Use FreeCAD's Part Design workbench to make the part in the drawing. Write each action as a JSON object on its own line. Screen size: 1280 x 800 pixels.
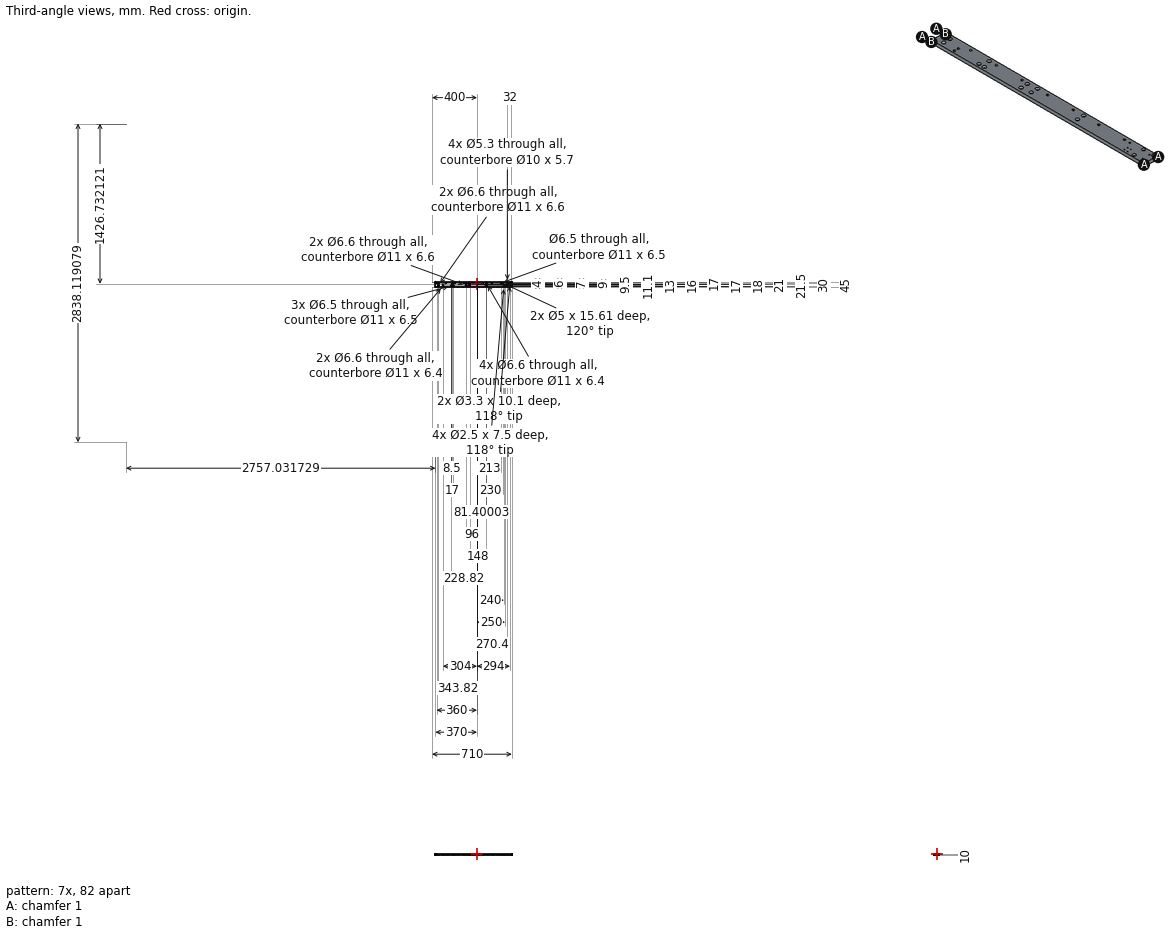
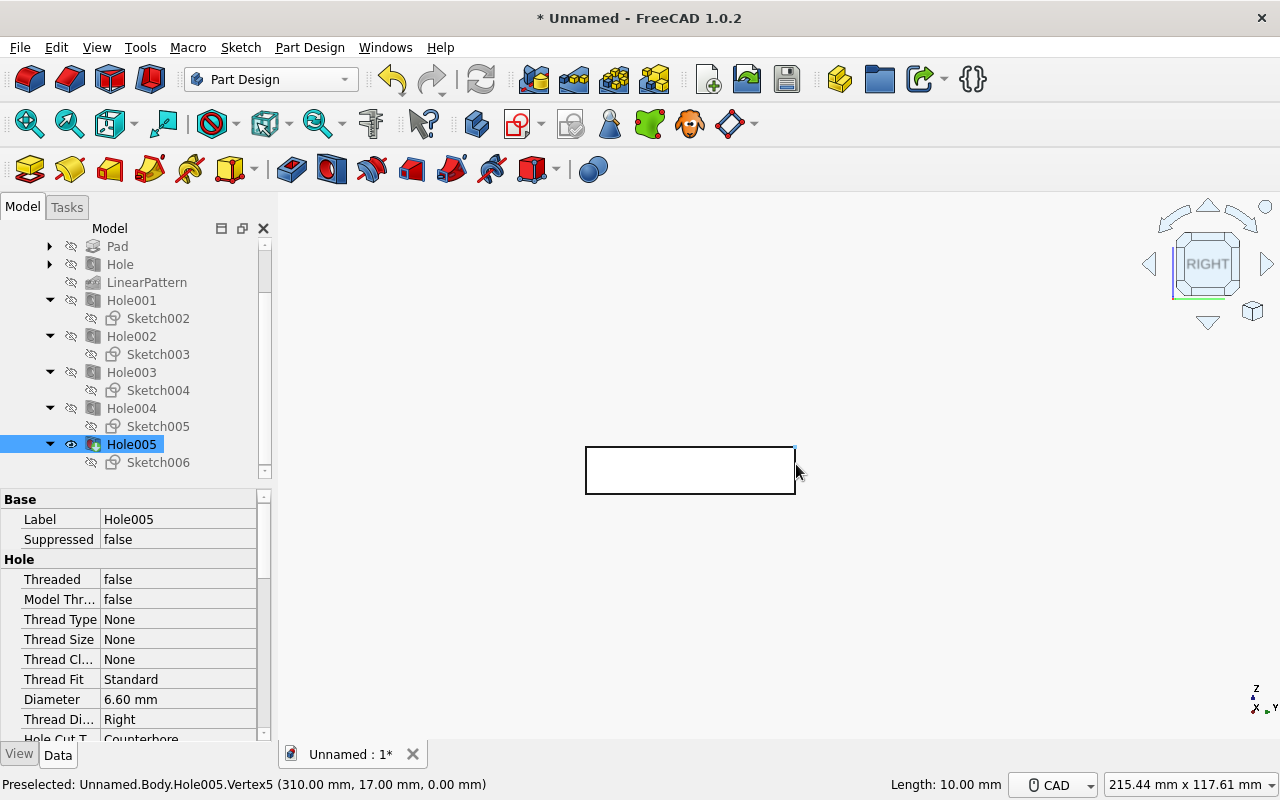
{"action": "left_click", "coordinate": [795, 470], "text": "ctrl"}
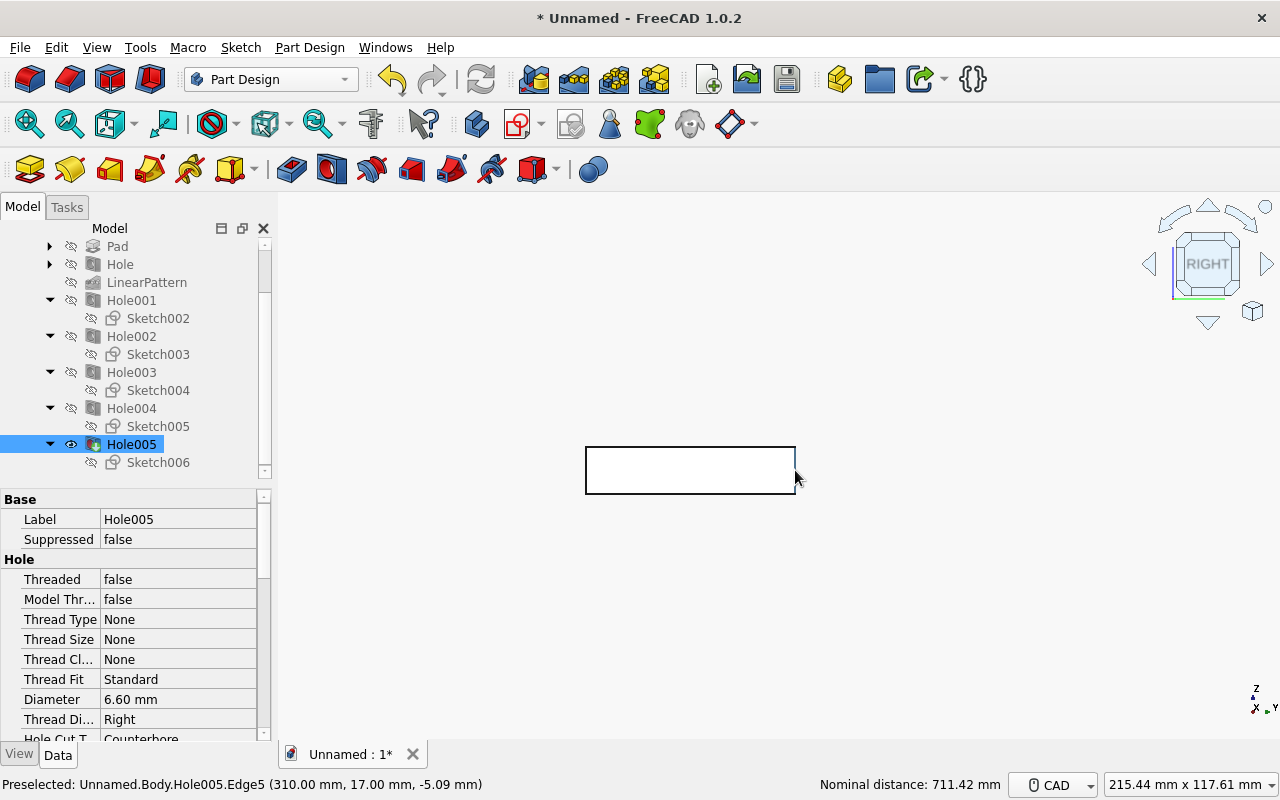
{"action": "left_click", "coordinate": [586, 470], "text": "ctrl"}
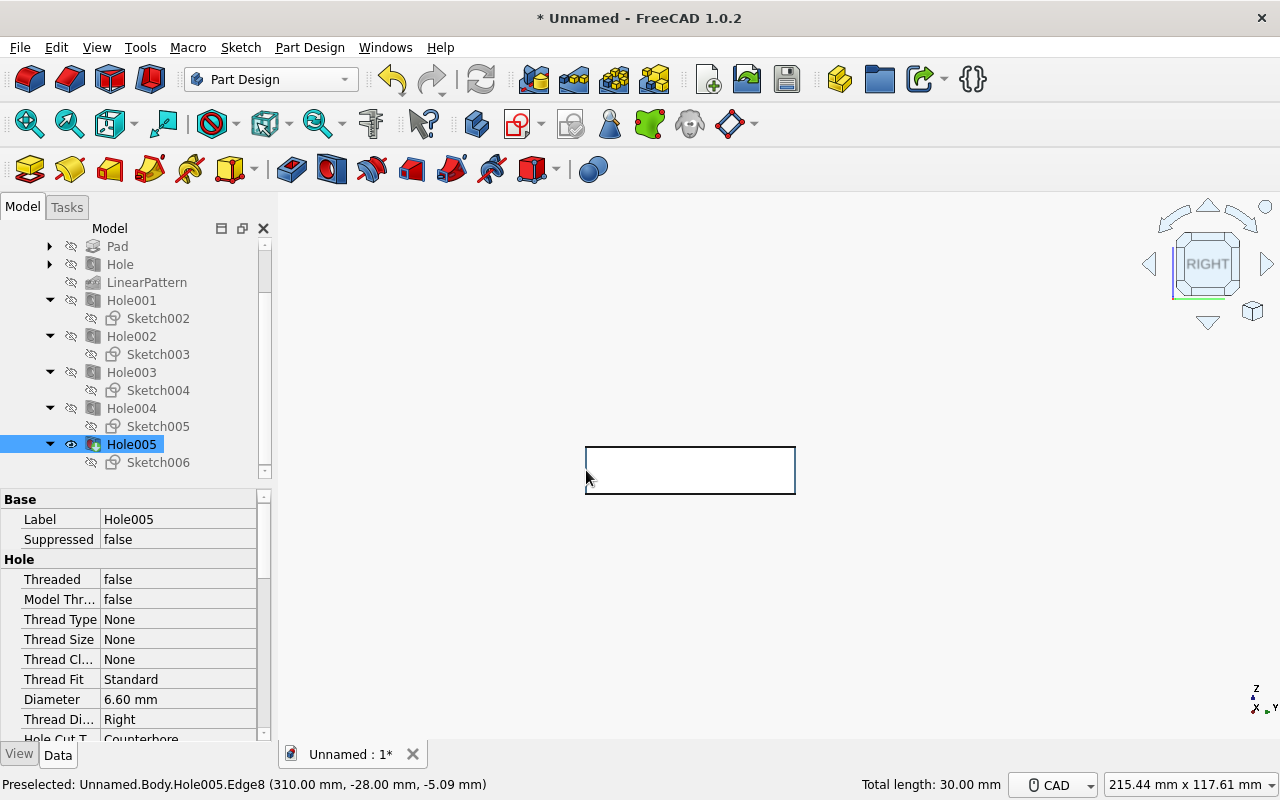
{"action": "left_click", "coordinate": [30, 124]}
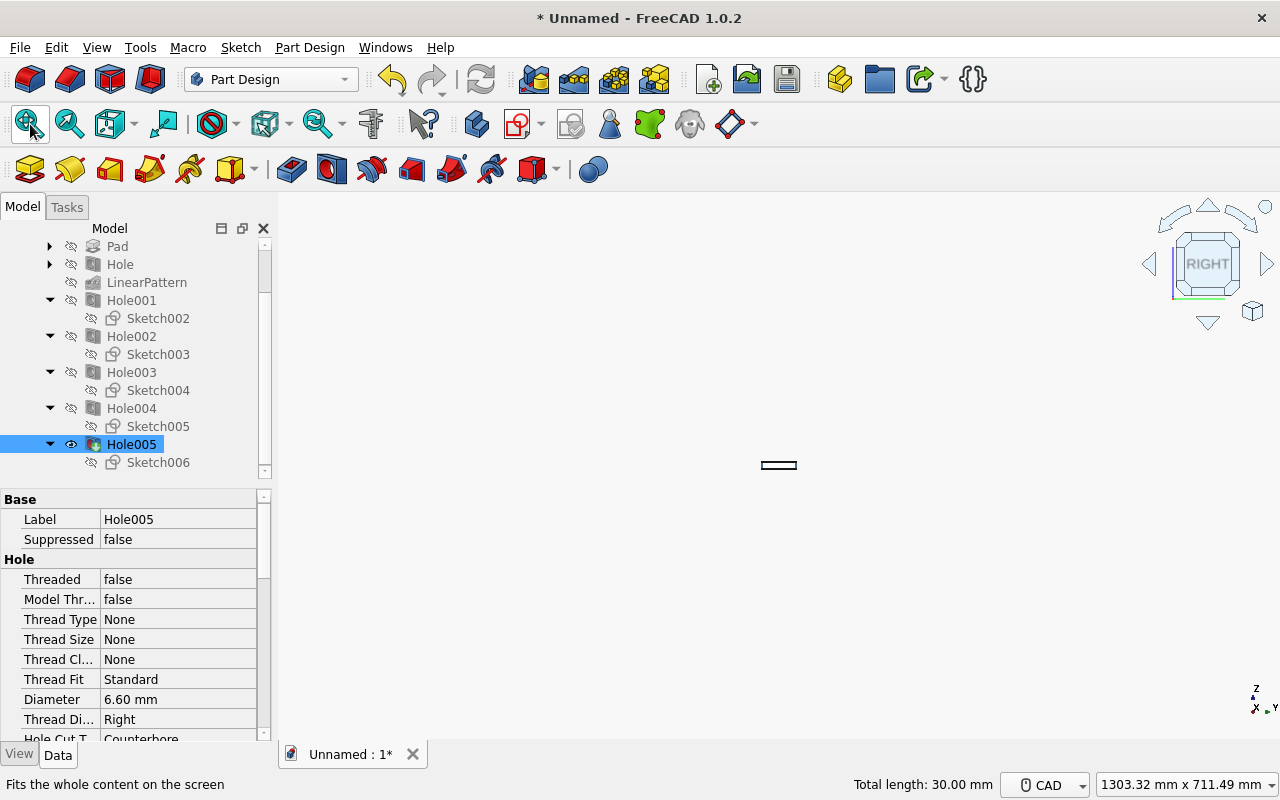
{"action": "key", "text": "5"}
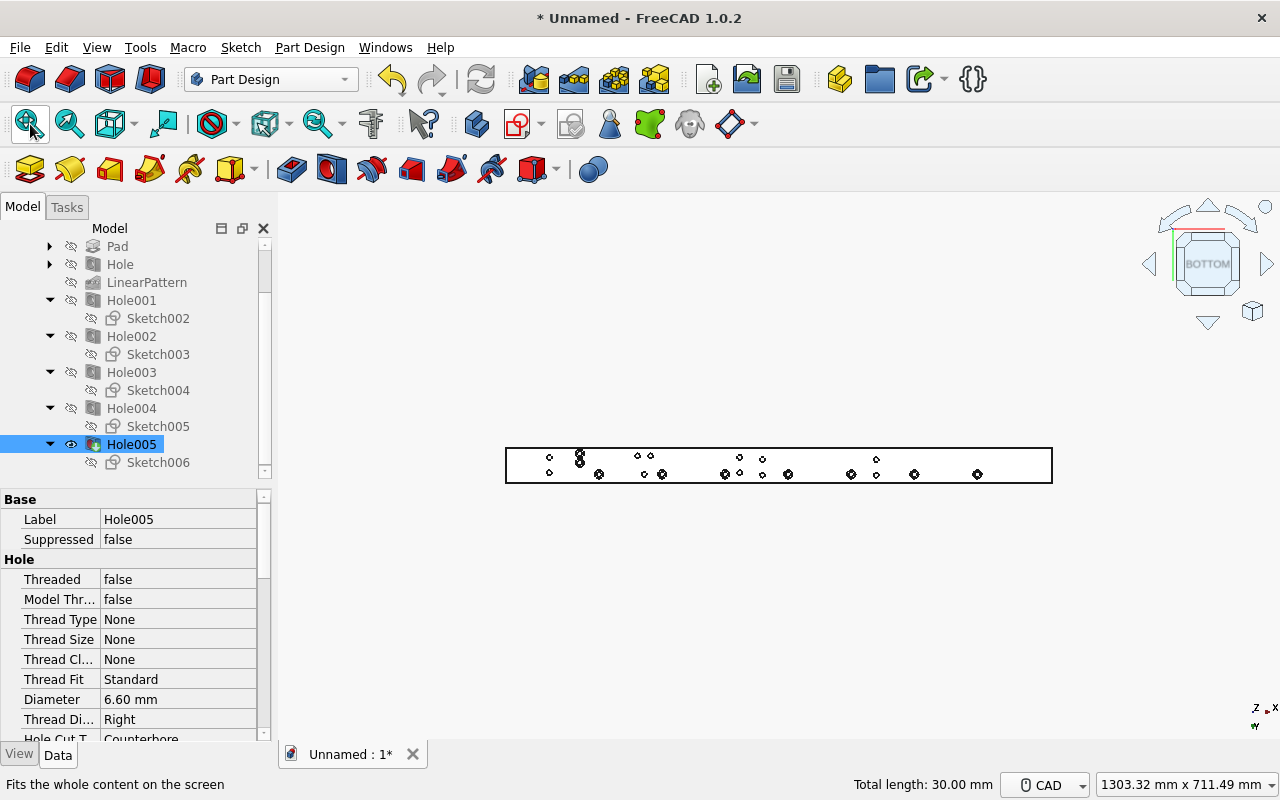
{"action": "scroll", "coordinate": [506, 482], "scroll_direction": "up", "scroll_amount": 9}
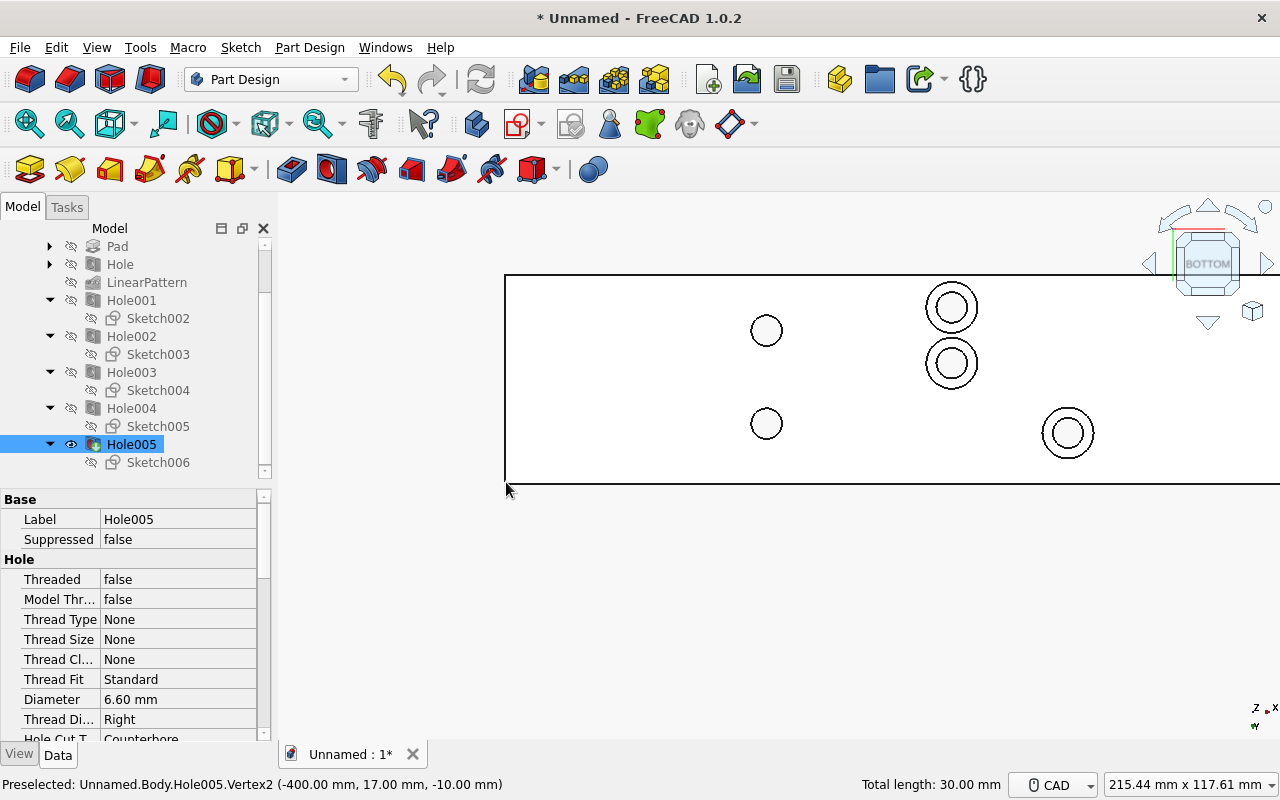
{"action": "left_click", "coordinate": [30, 124]}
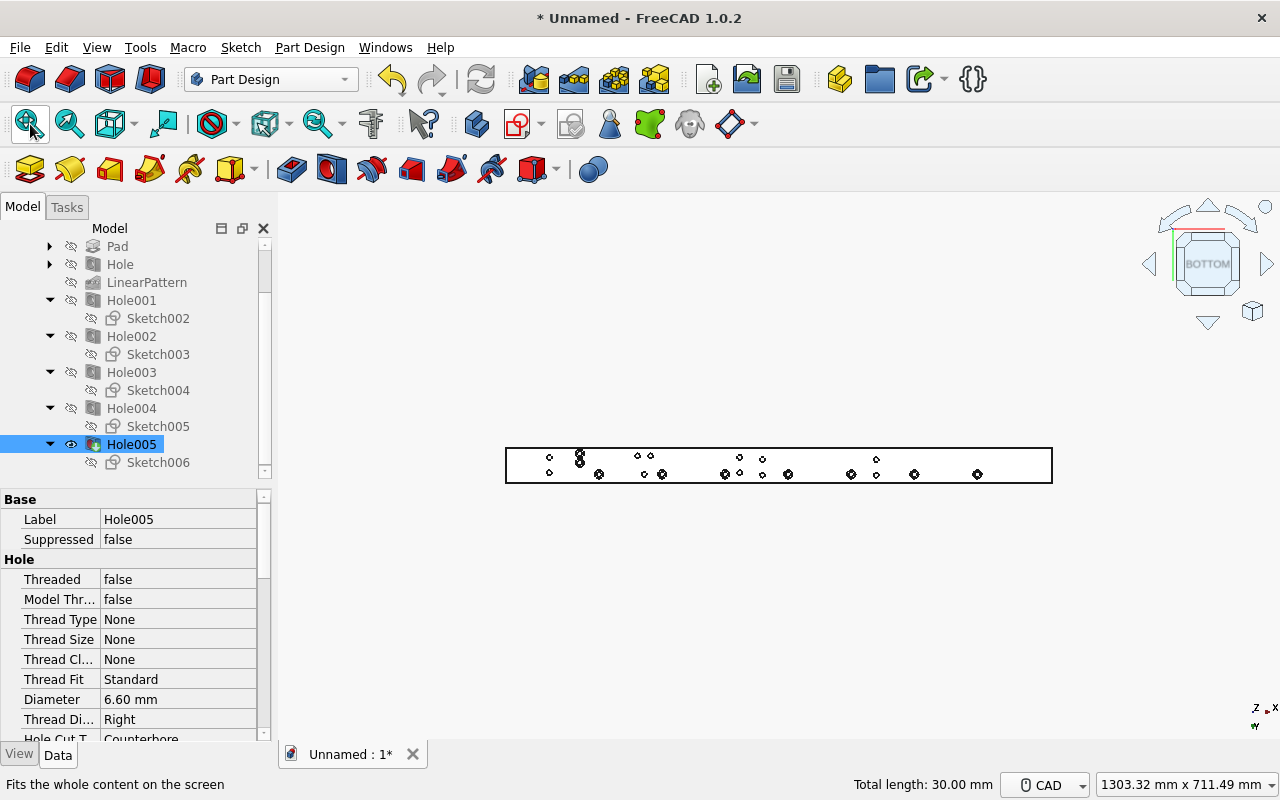
{"action": "key", "text": "4"}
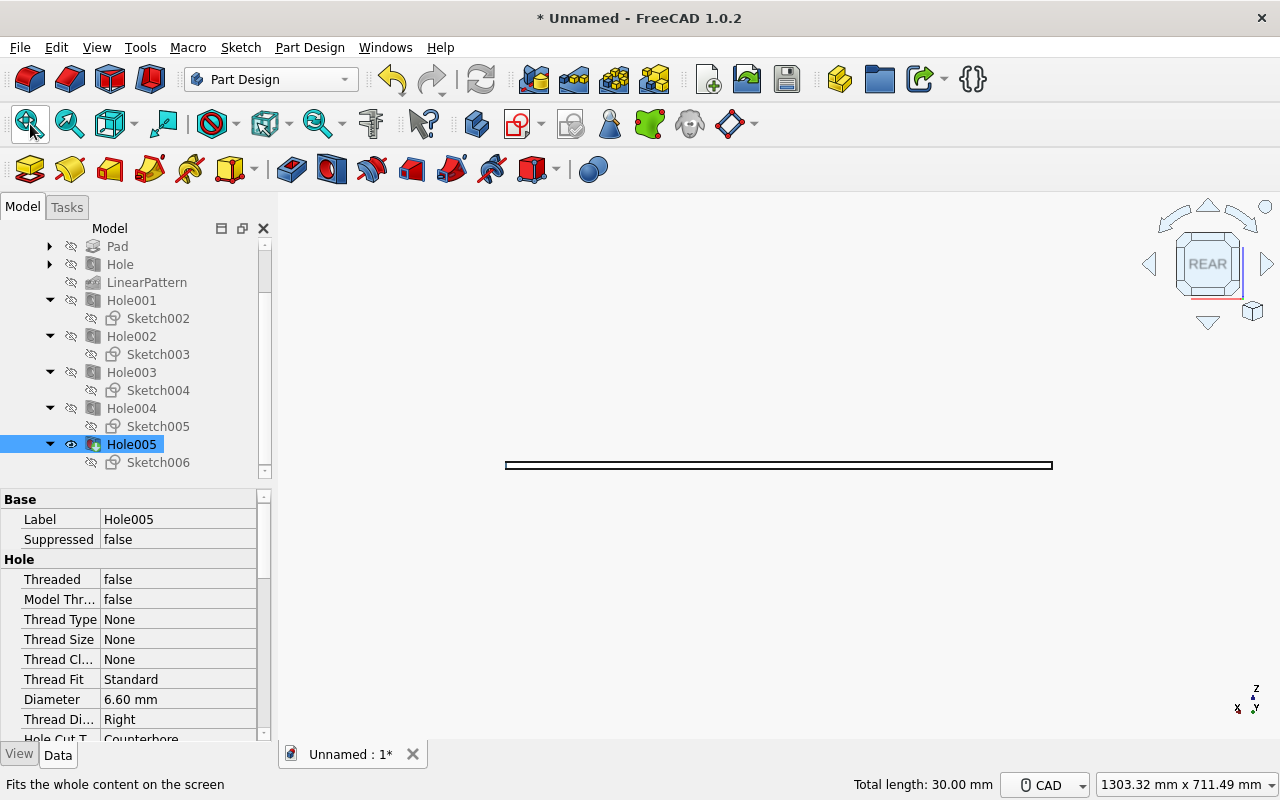
{"action": "scroll", "coordinate": [1052, 465], "scroll_direction": "up", "scroll_amount": 9}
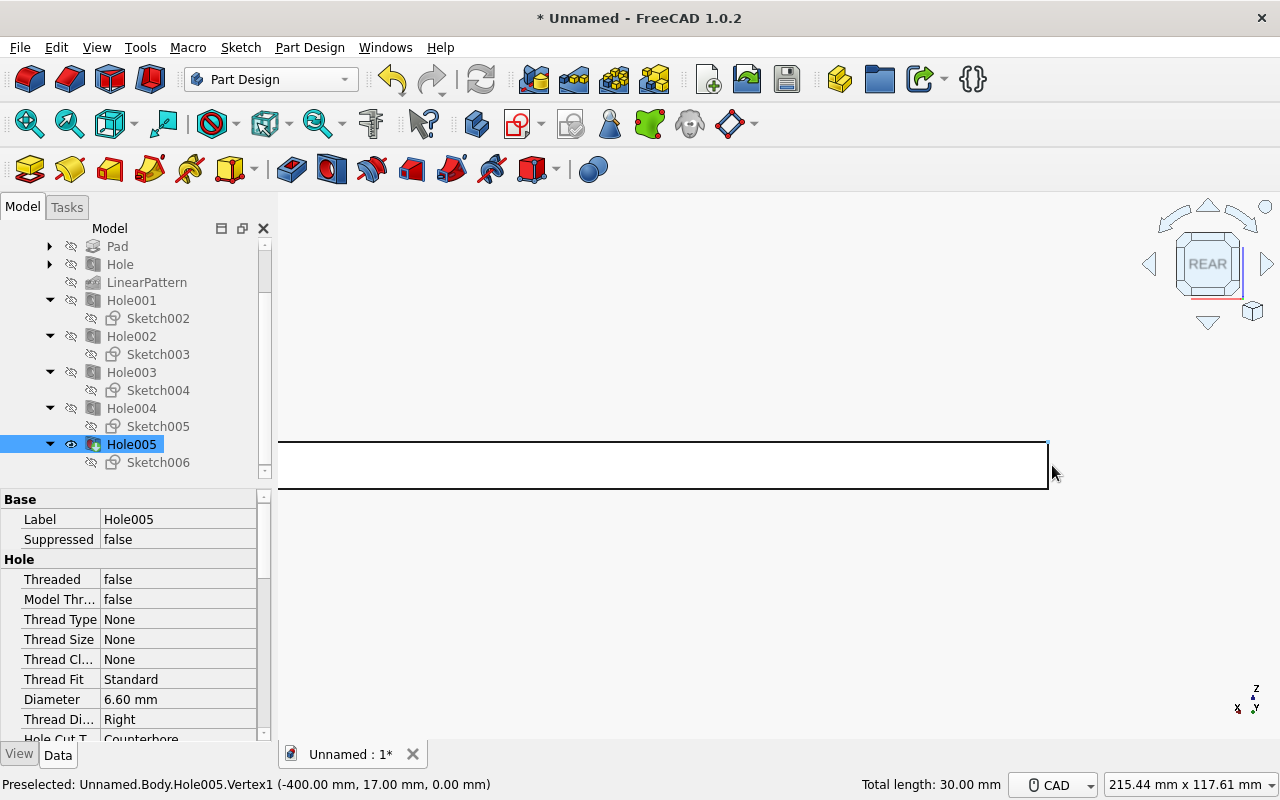
{"action": "left_click", "coordinate": [1048, 465], "text": "ctrl"}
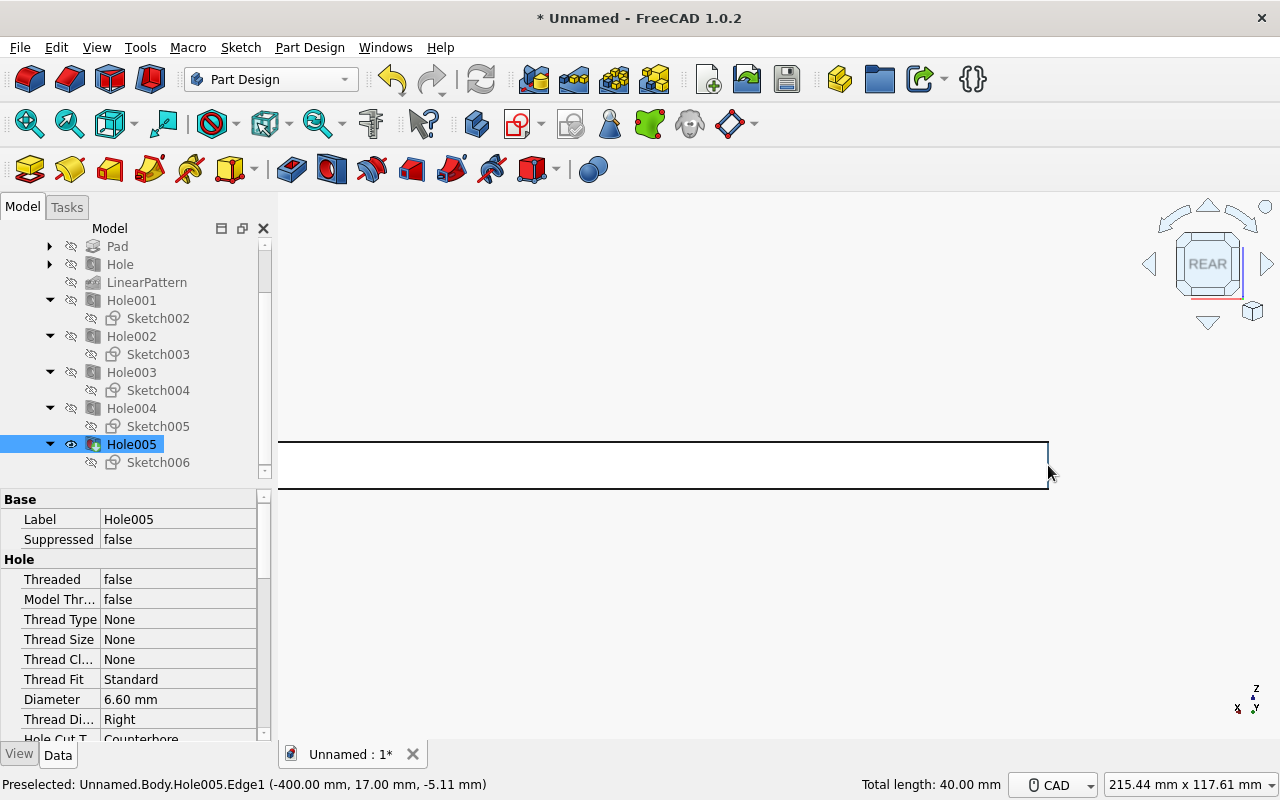
{"action": "left_click", "coordinate": [70, 80]}